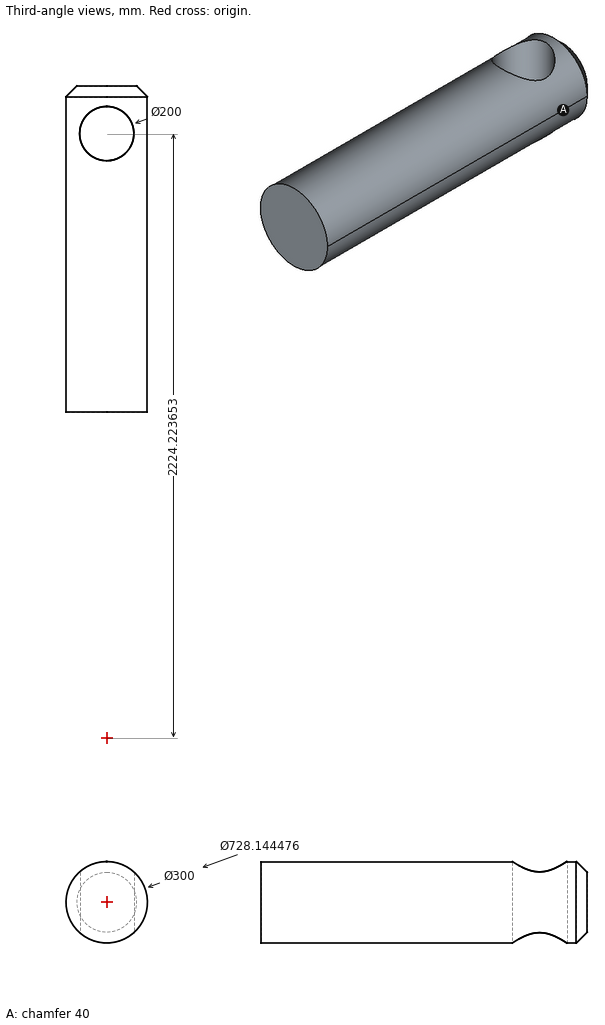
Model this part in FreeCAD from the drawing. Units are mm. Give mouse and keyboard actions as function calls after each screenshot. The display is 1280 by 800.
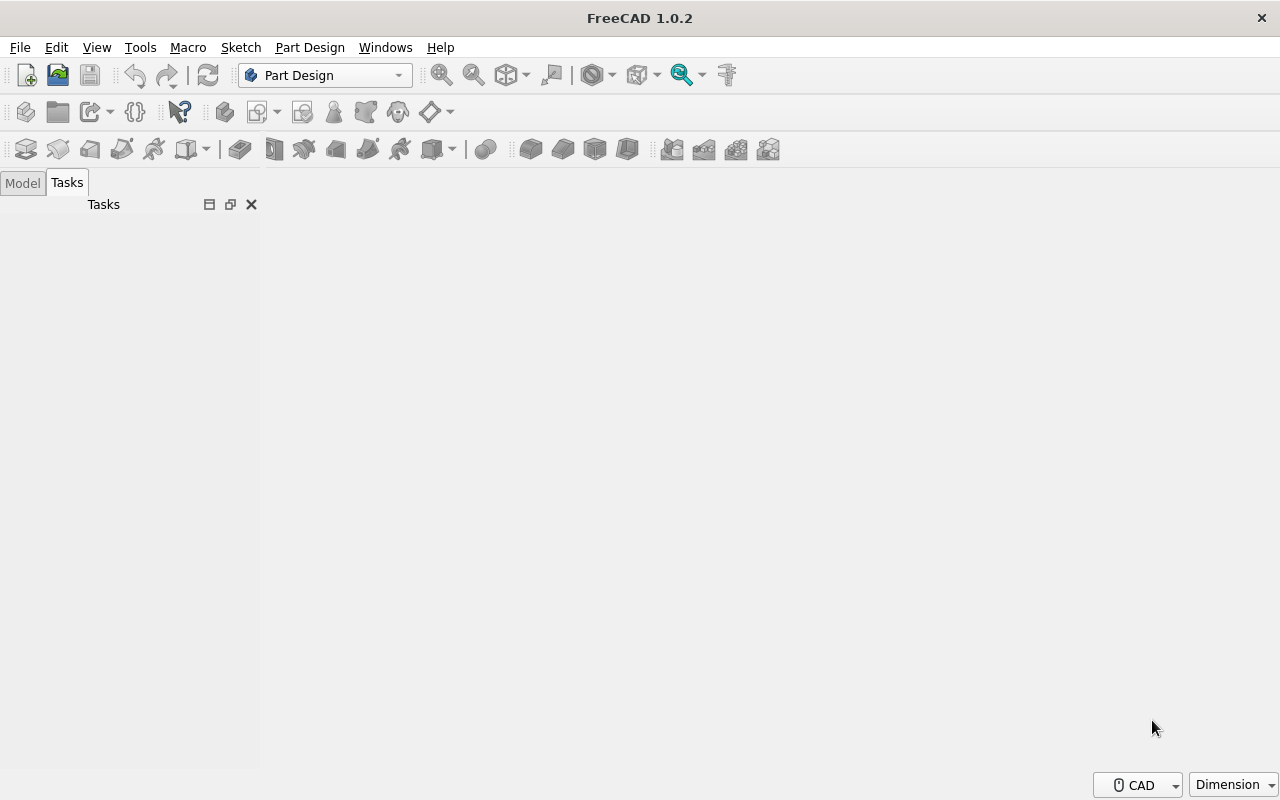
click(344, 112)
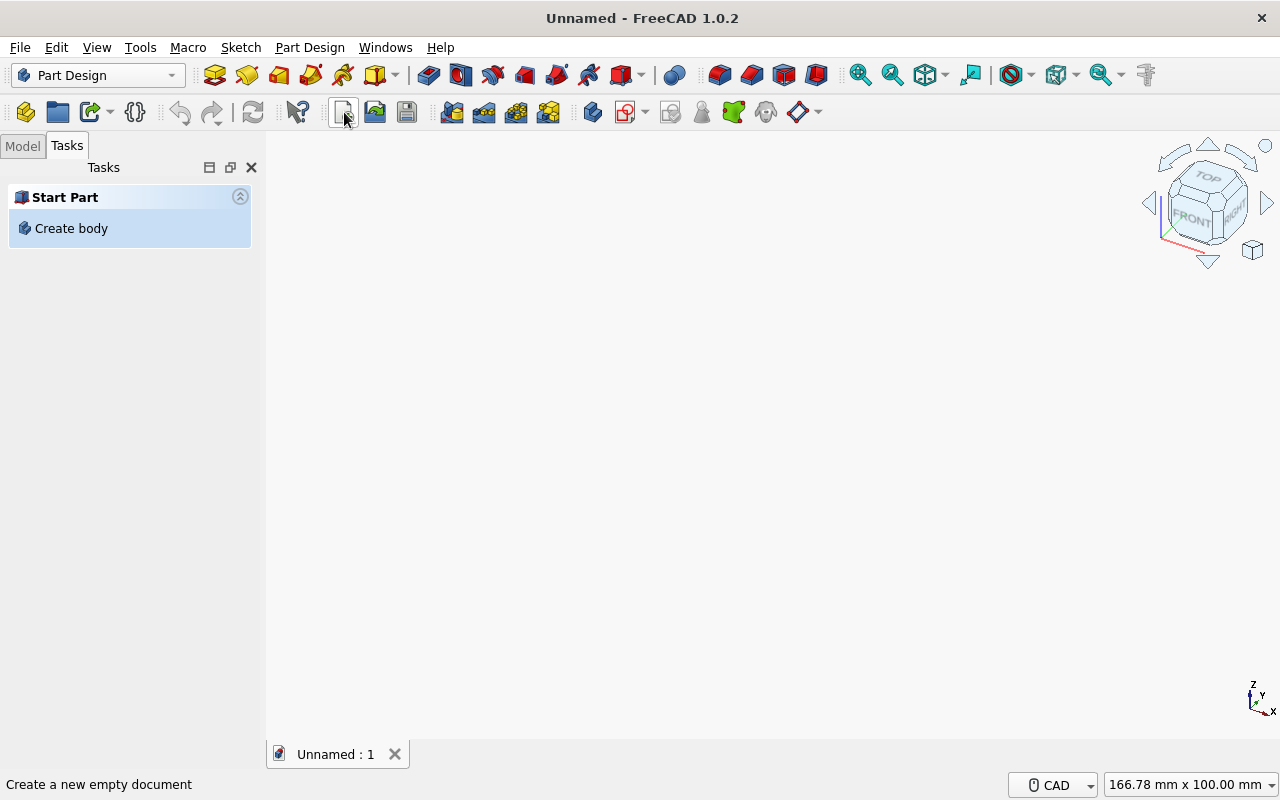
click(626, 112)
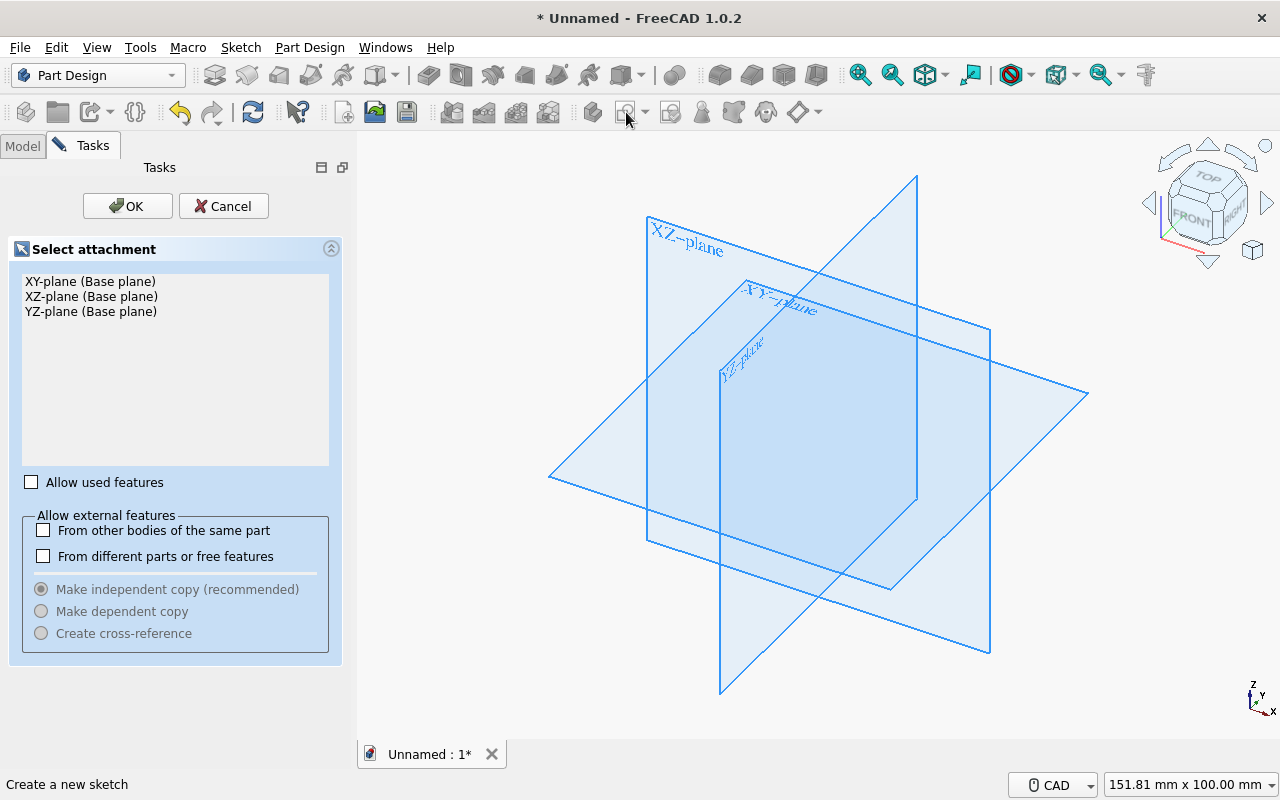
click(82, 296)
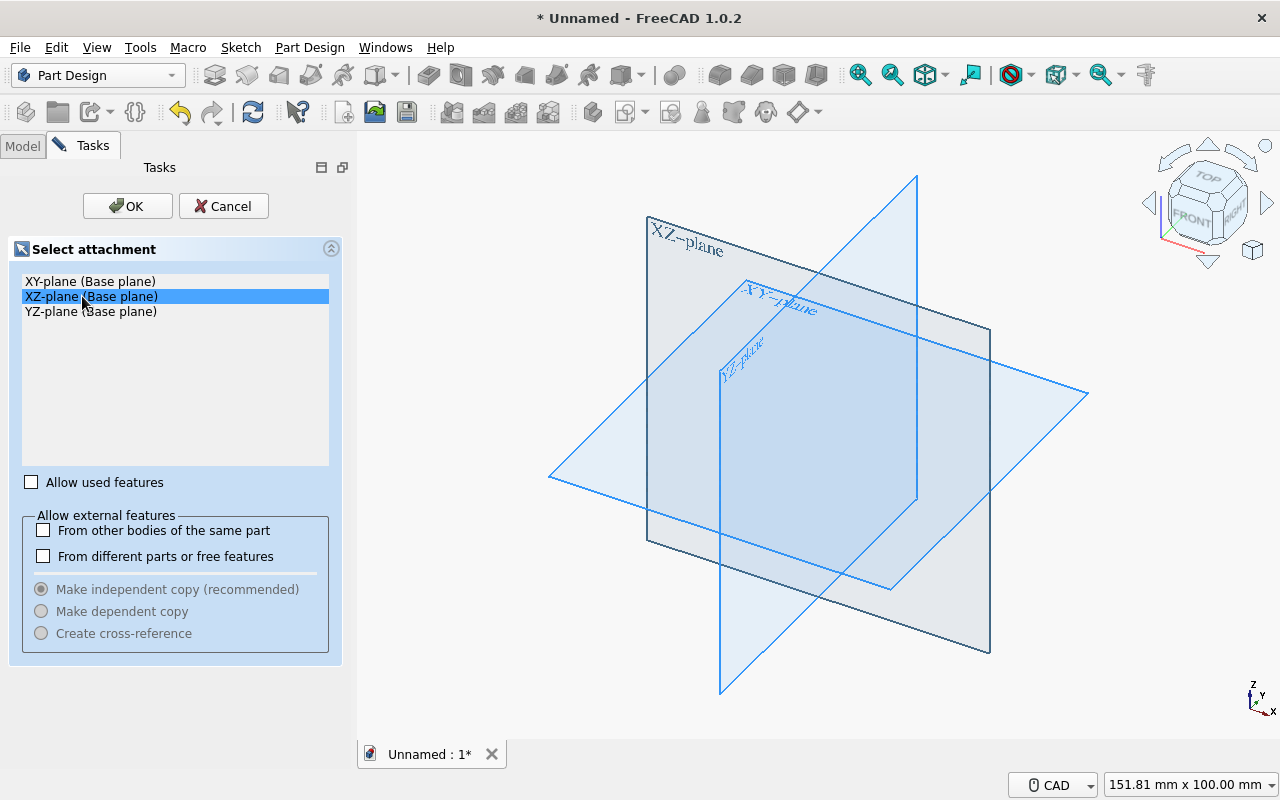
click(128, 206)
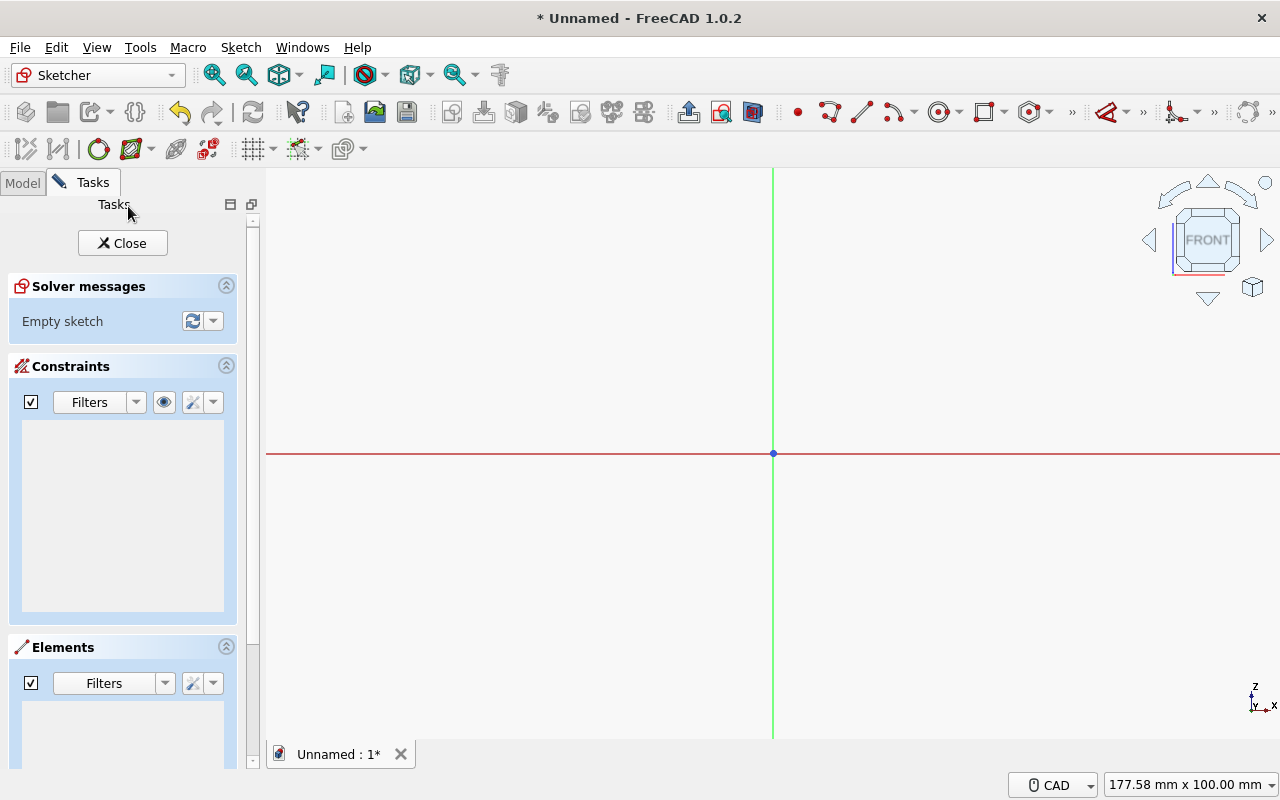
scroll(687, 454, down, 8)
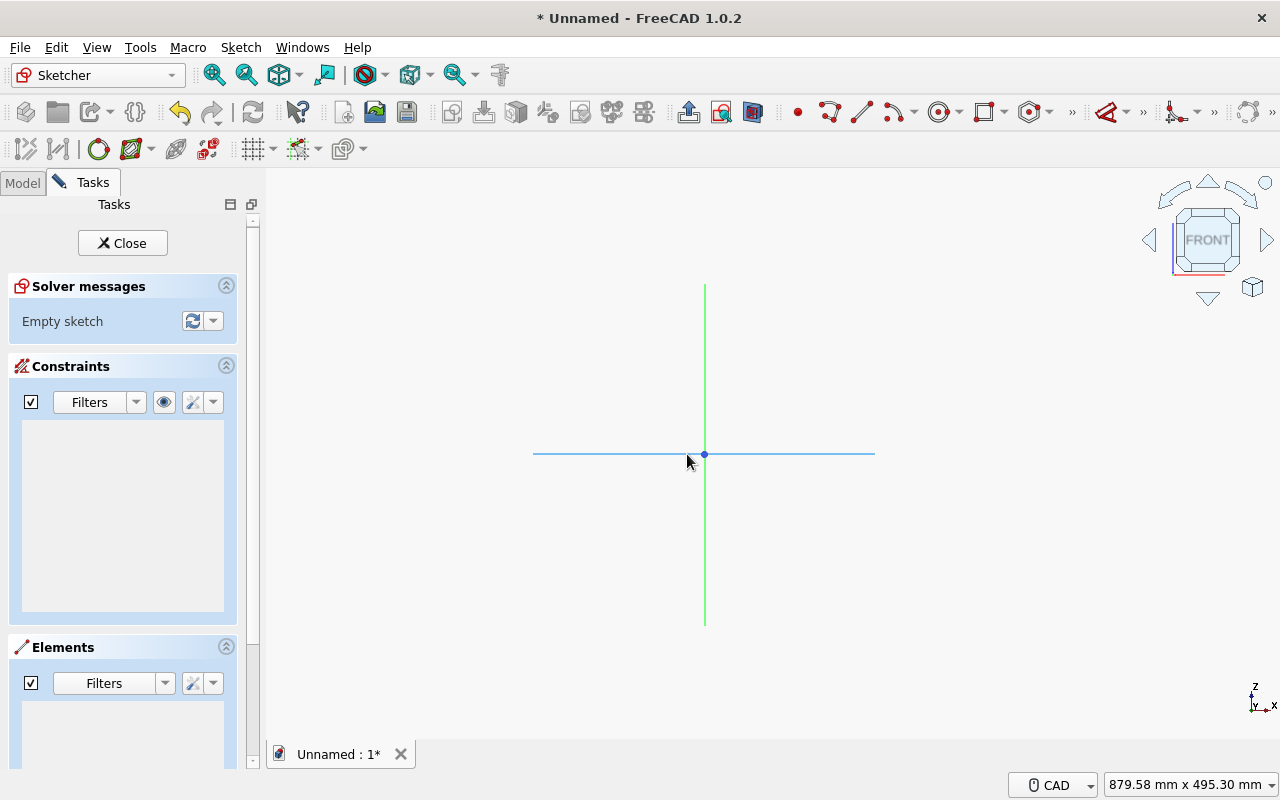
click(940, 112)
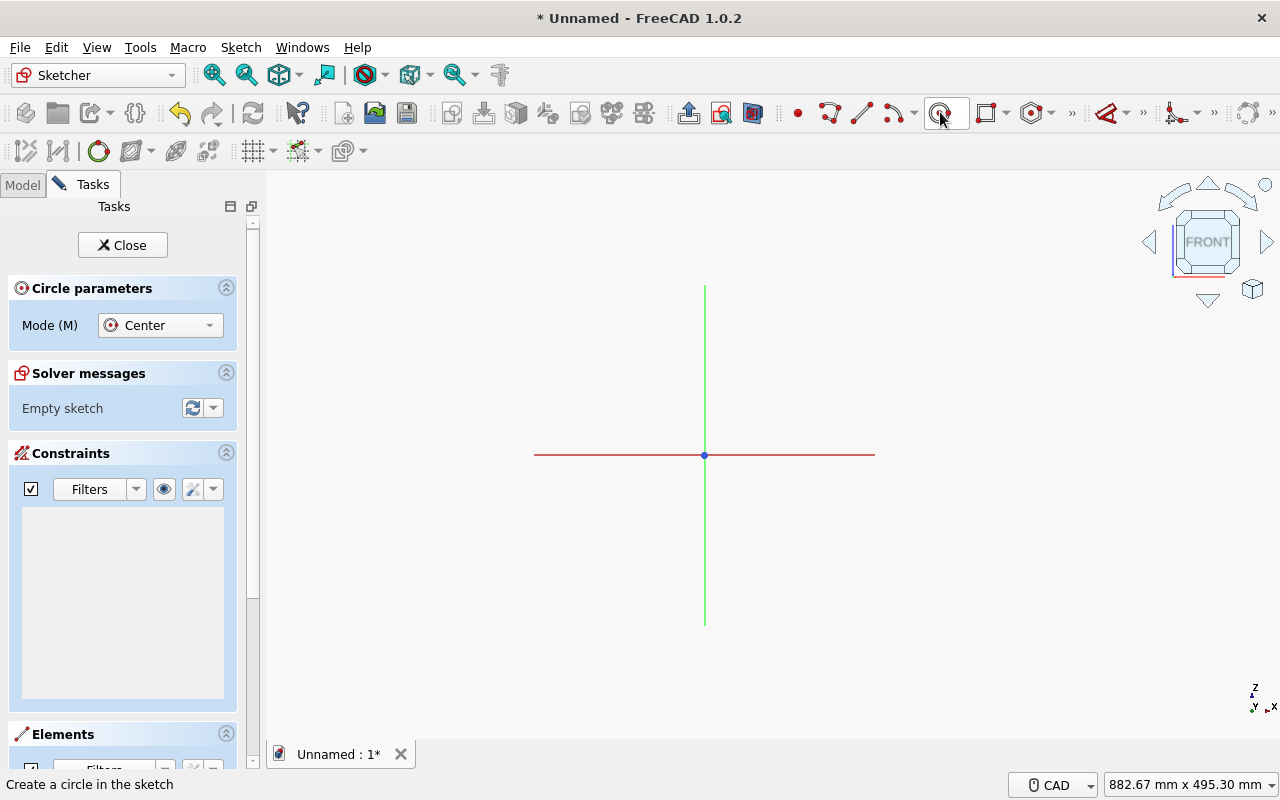
click(705, 455)
move(827, 333)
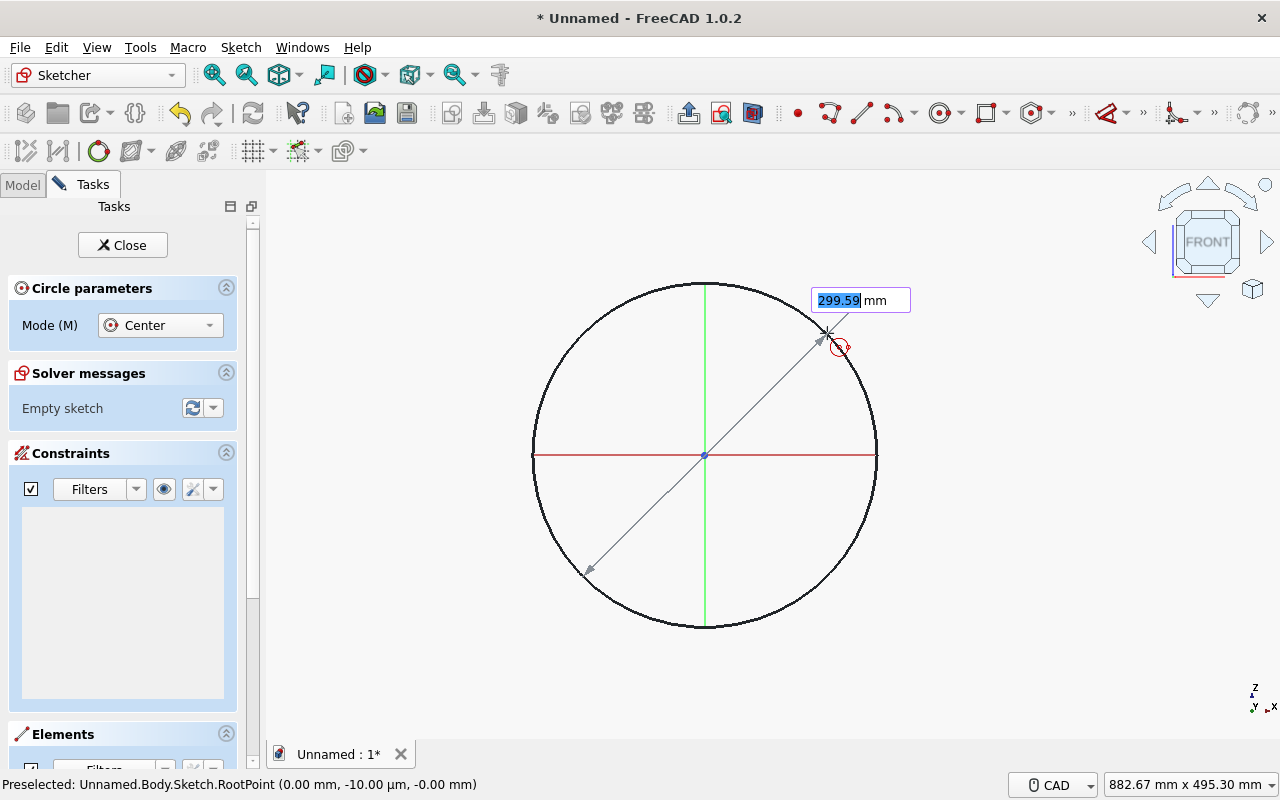
text(300)
key(Return)
key(Escape)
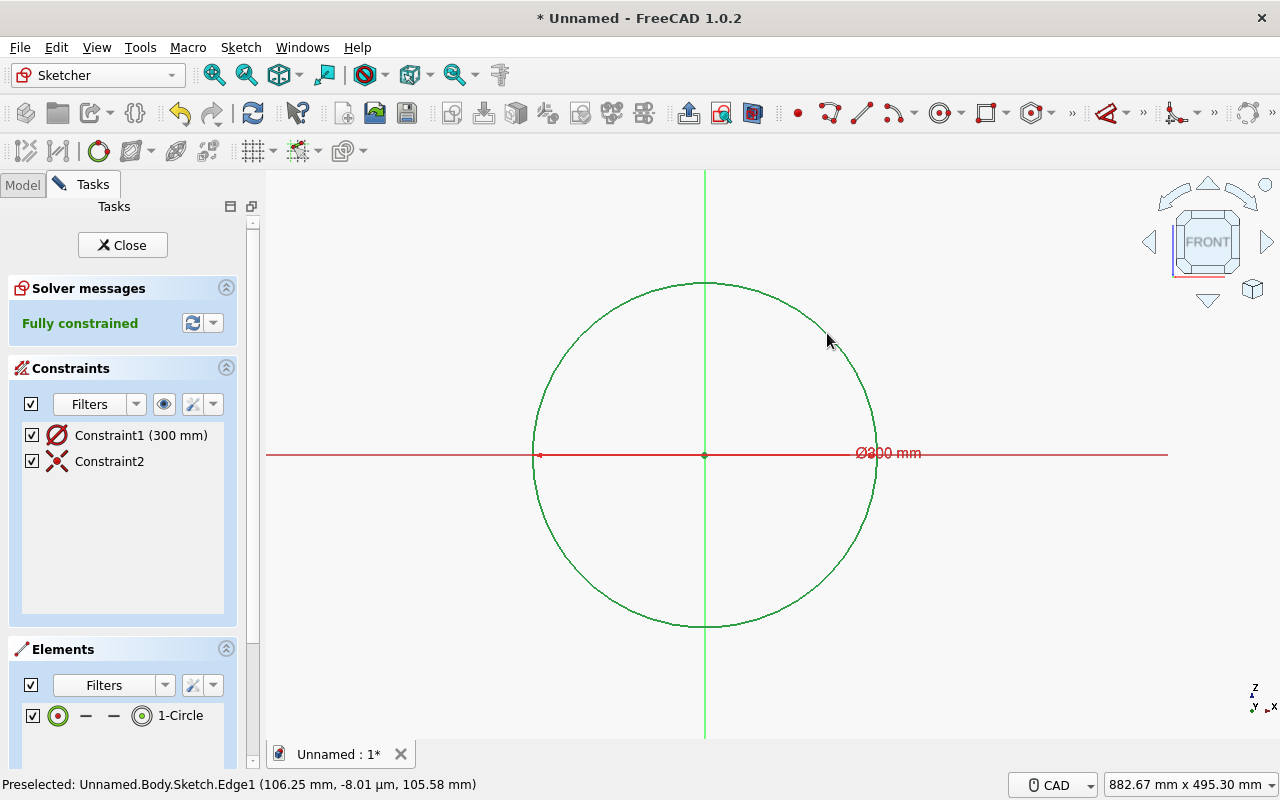
click(123, 245)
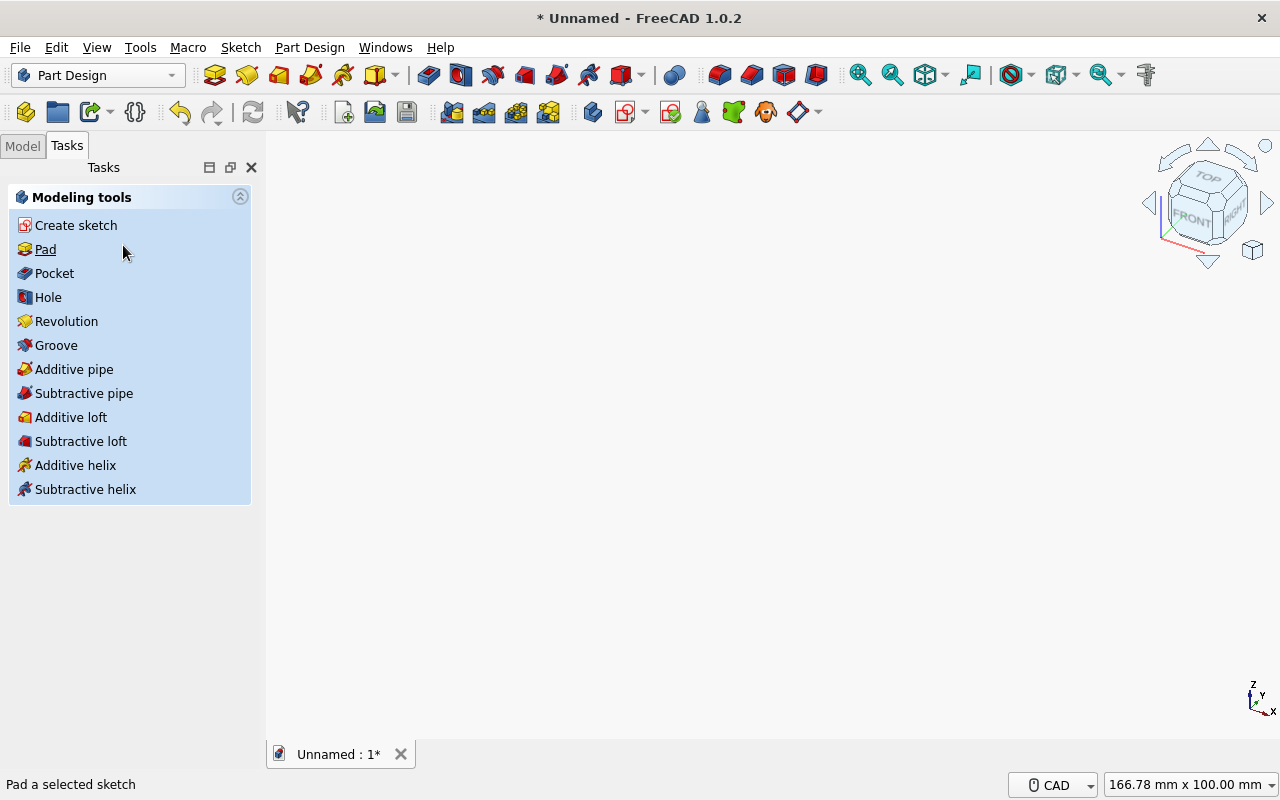
click(216, 76)